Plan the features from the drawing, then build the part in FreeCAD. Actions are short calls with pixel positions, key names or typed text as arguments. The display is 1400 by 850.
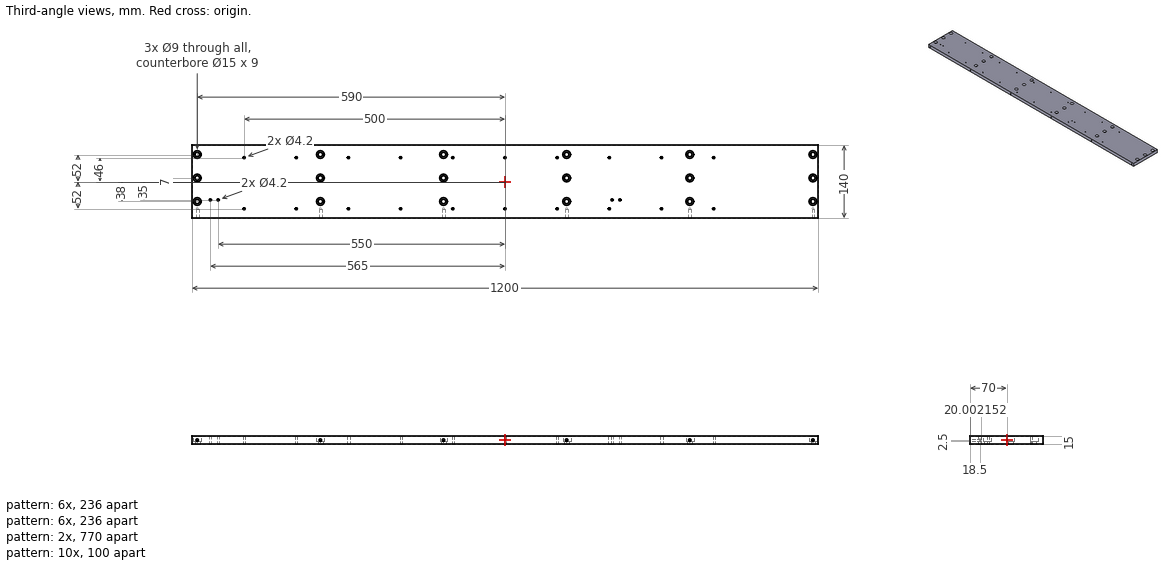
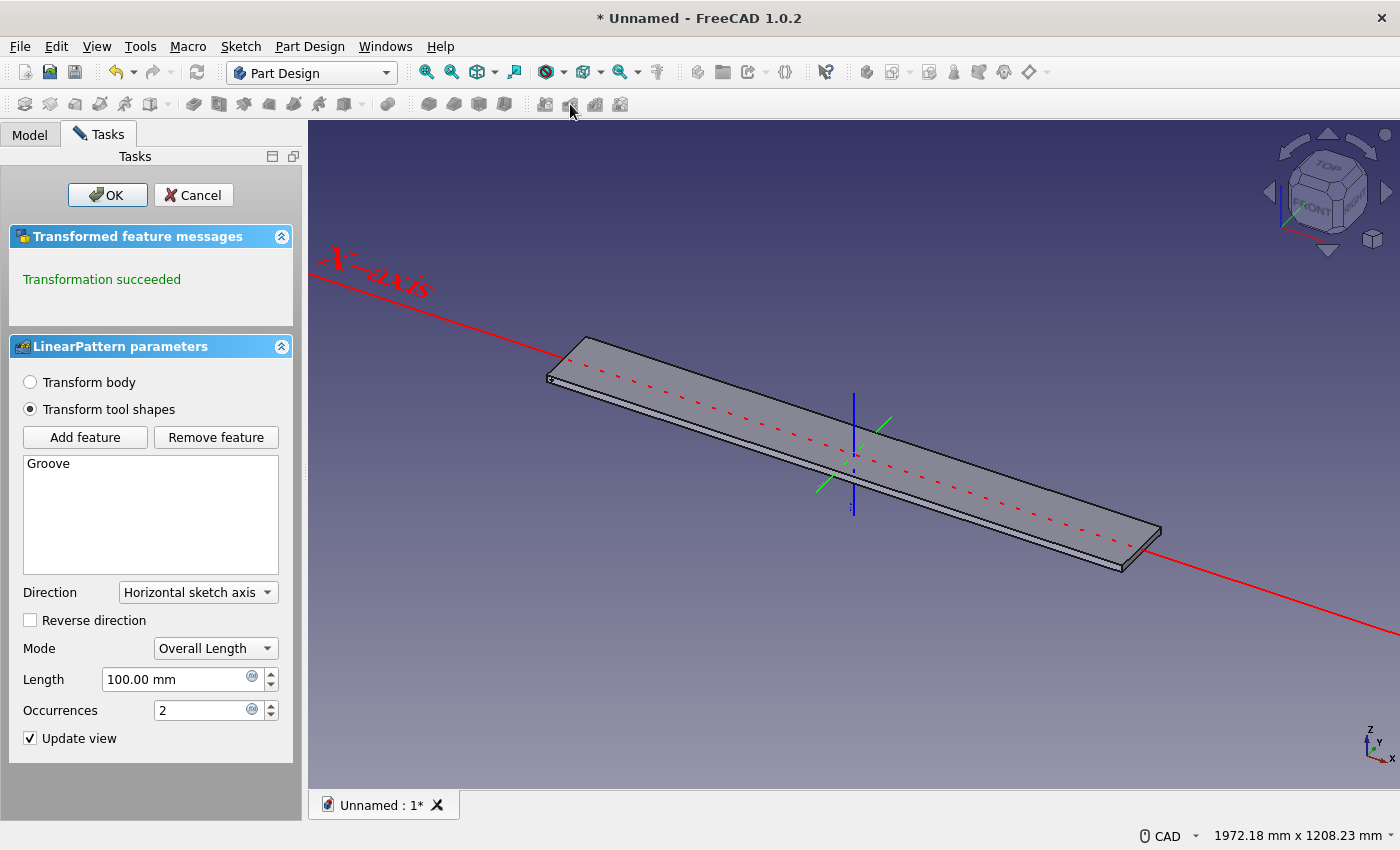
click(199, 592)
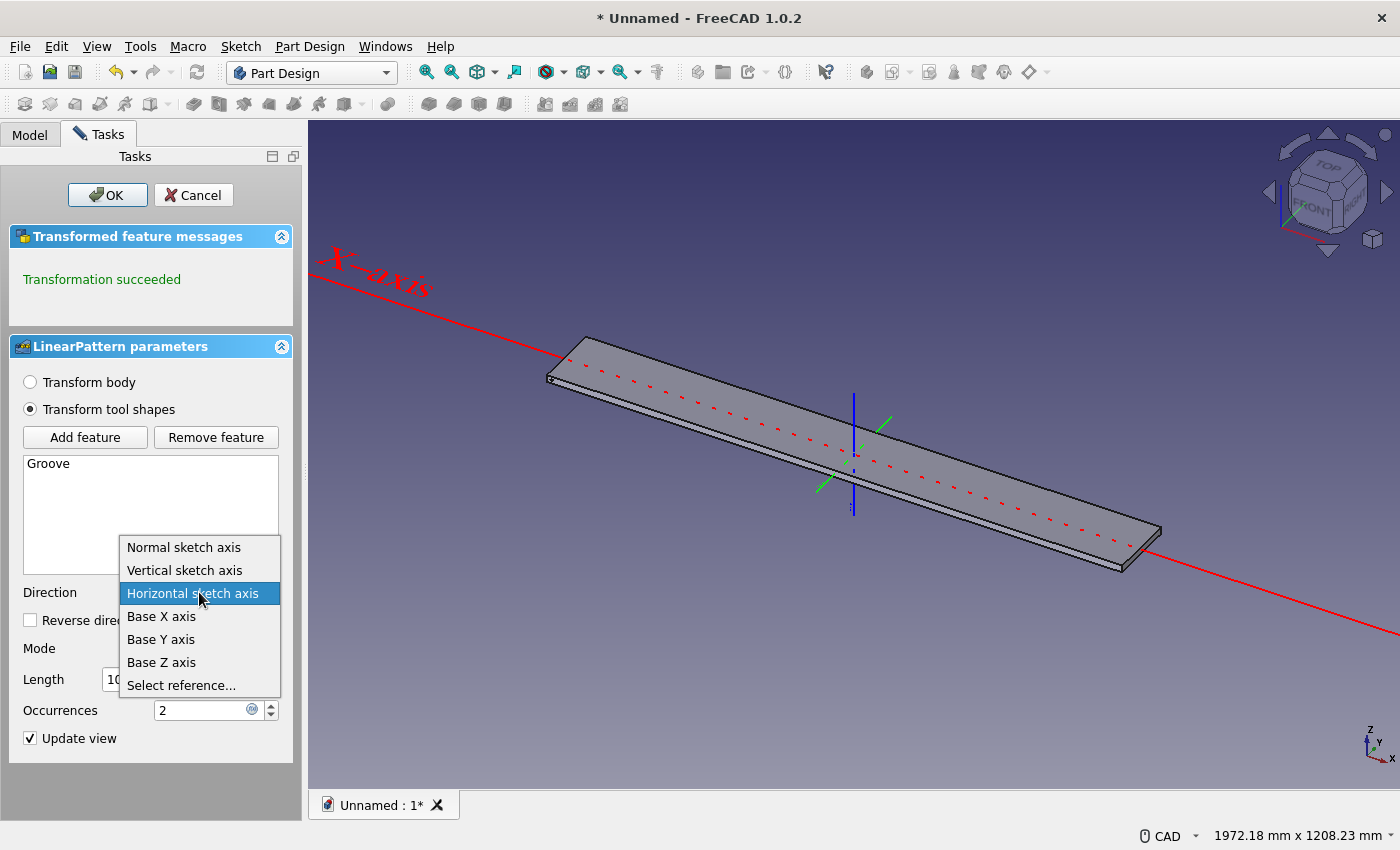
click(198, 616)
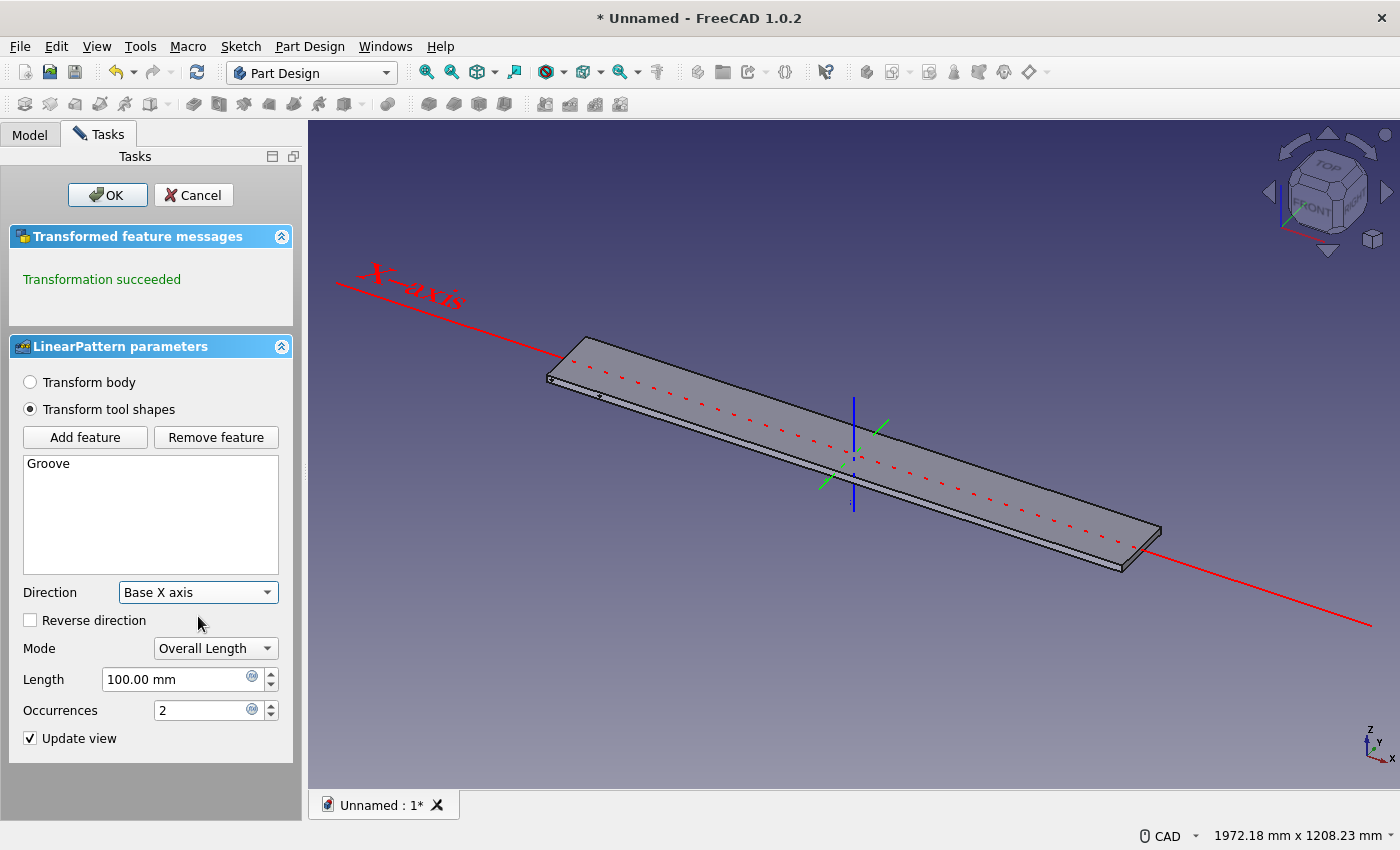
click(216, 648)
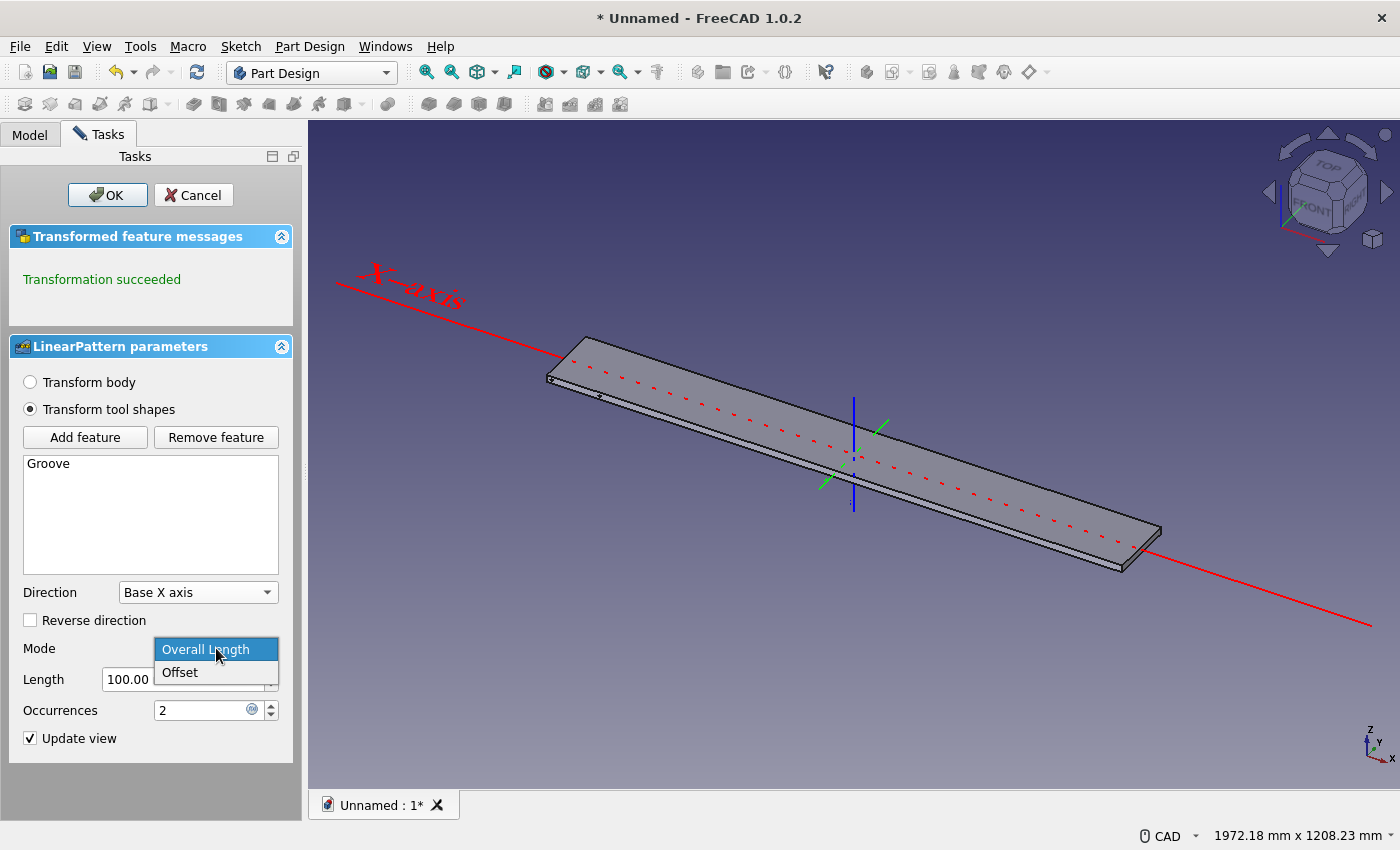
click(214, 672)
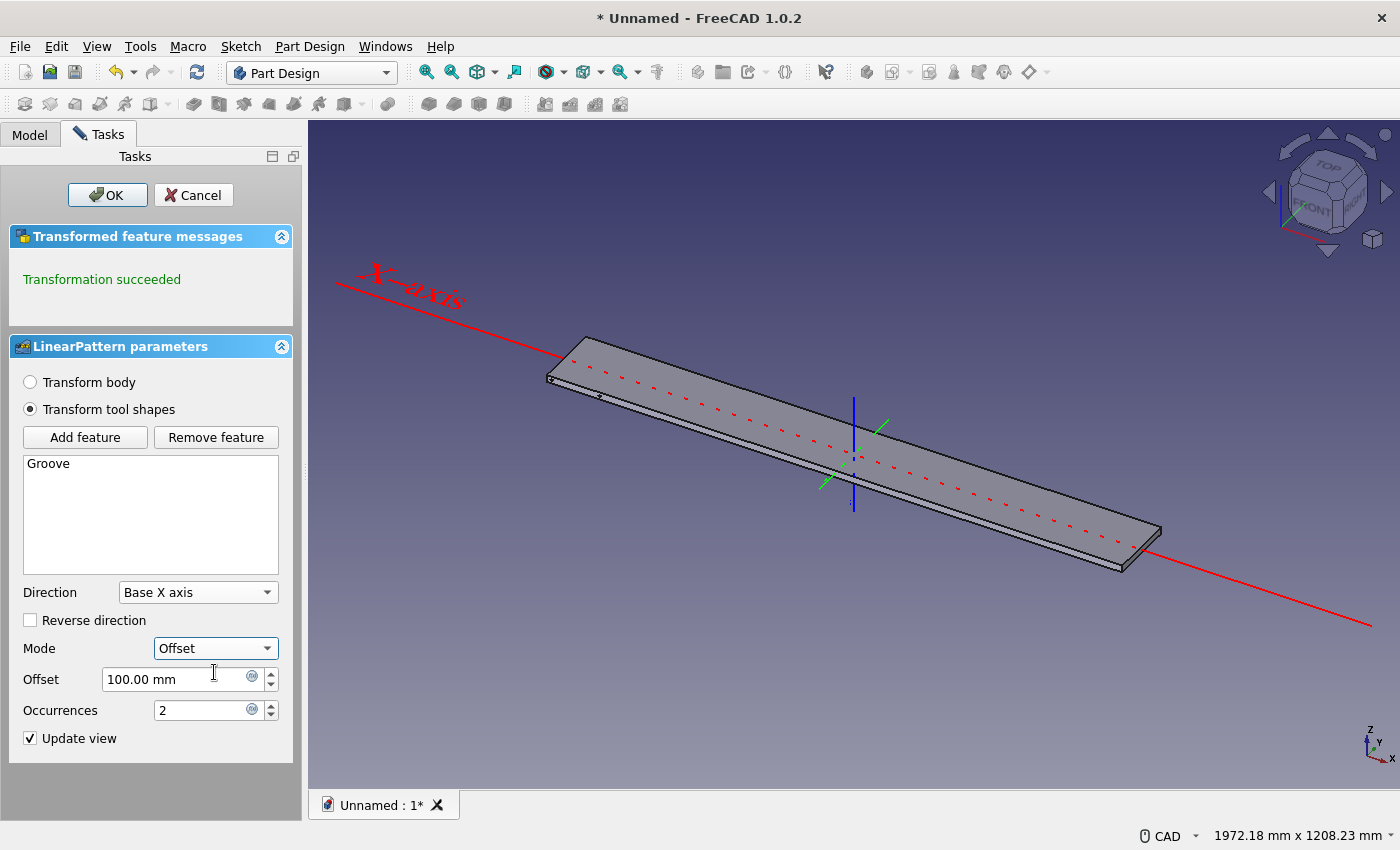
triple_click(184, 680)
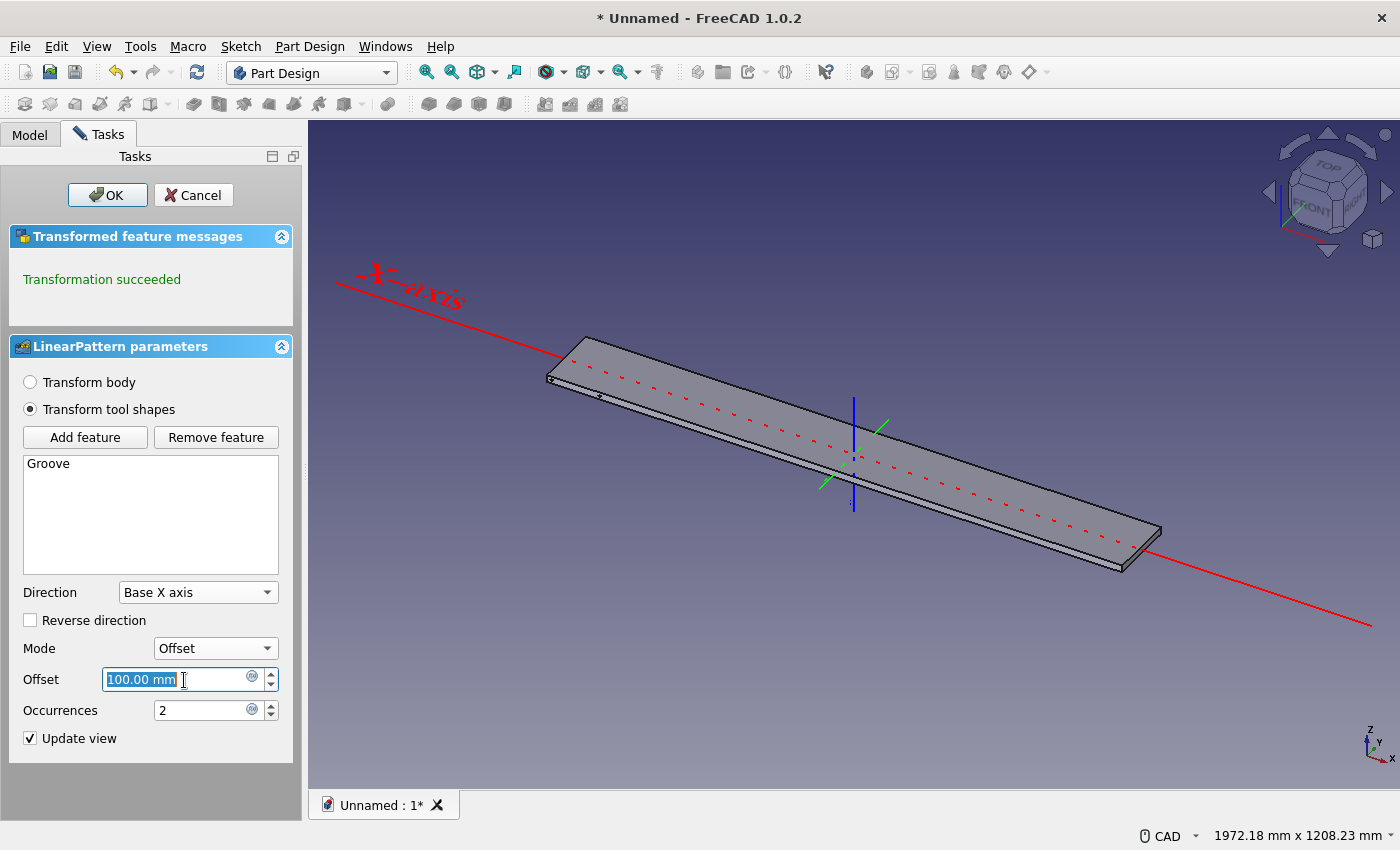
text(236)
key(Tab)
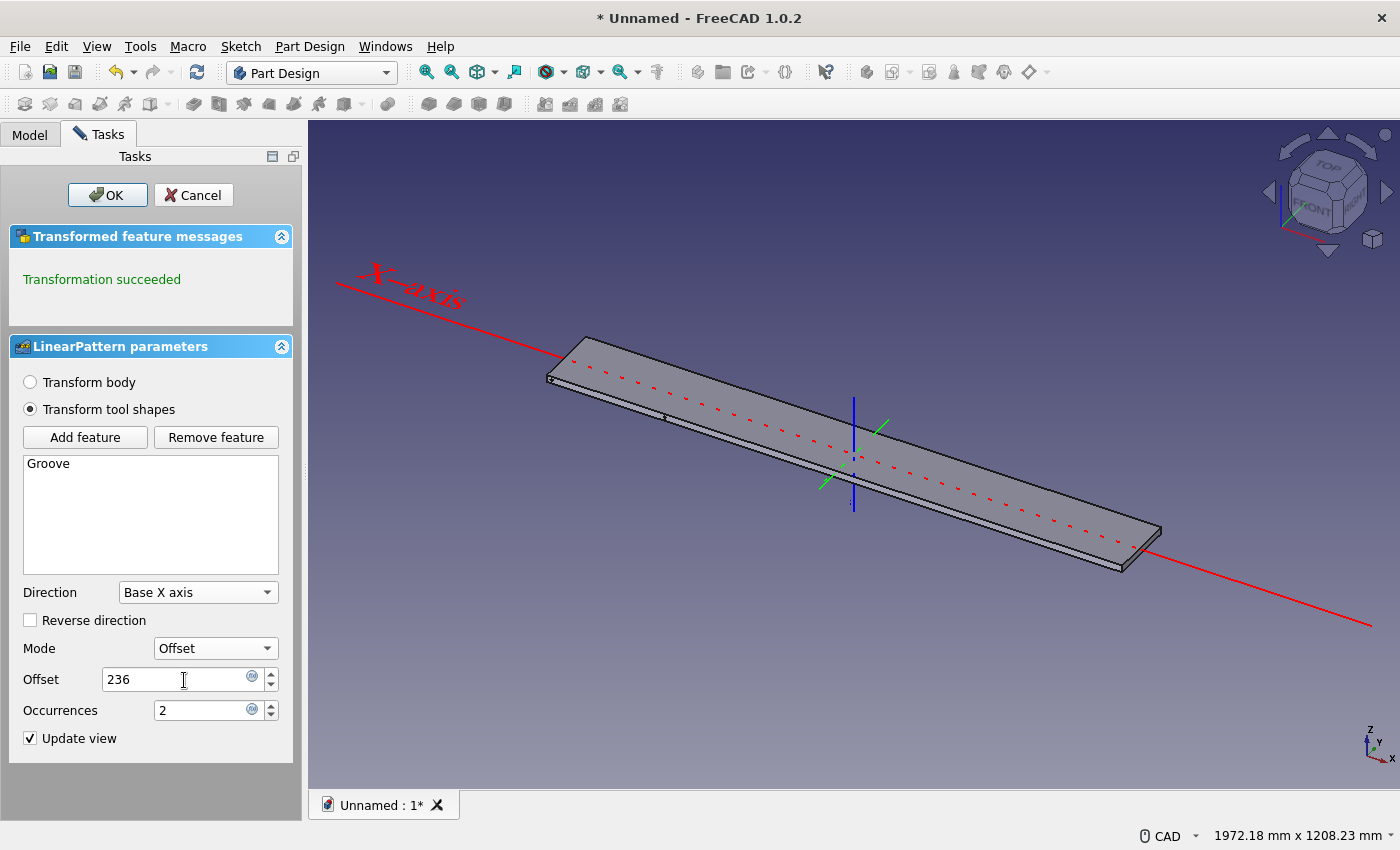
triple_click(210, 710)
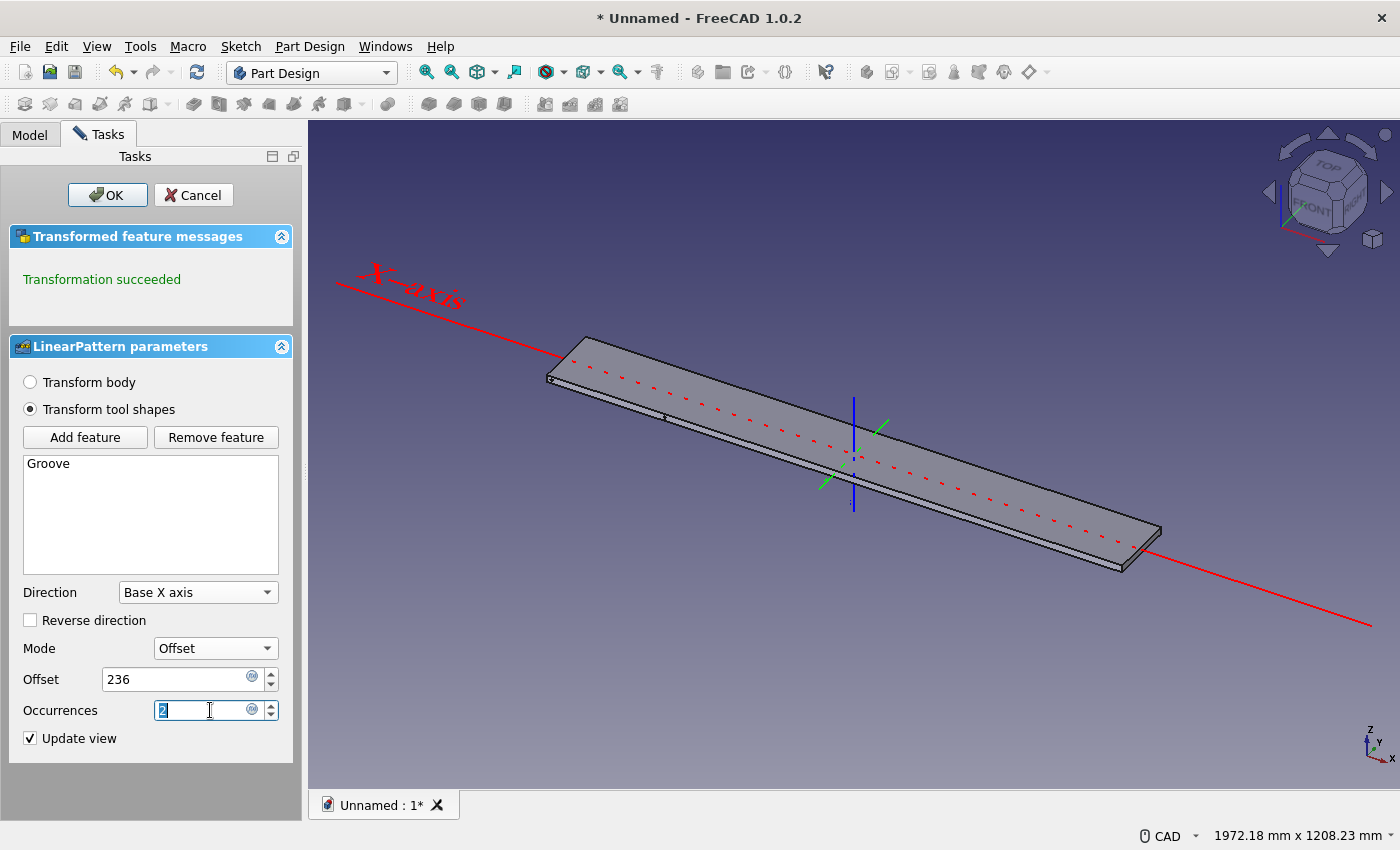
text(6)
key(Tab)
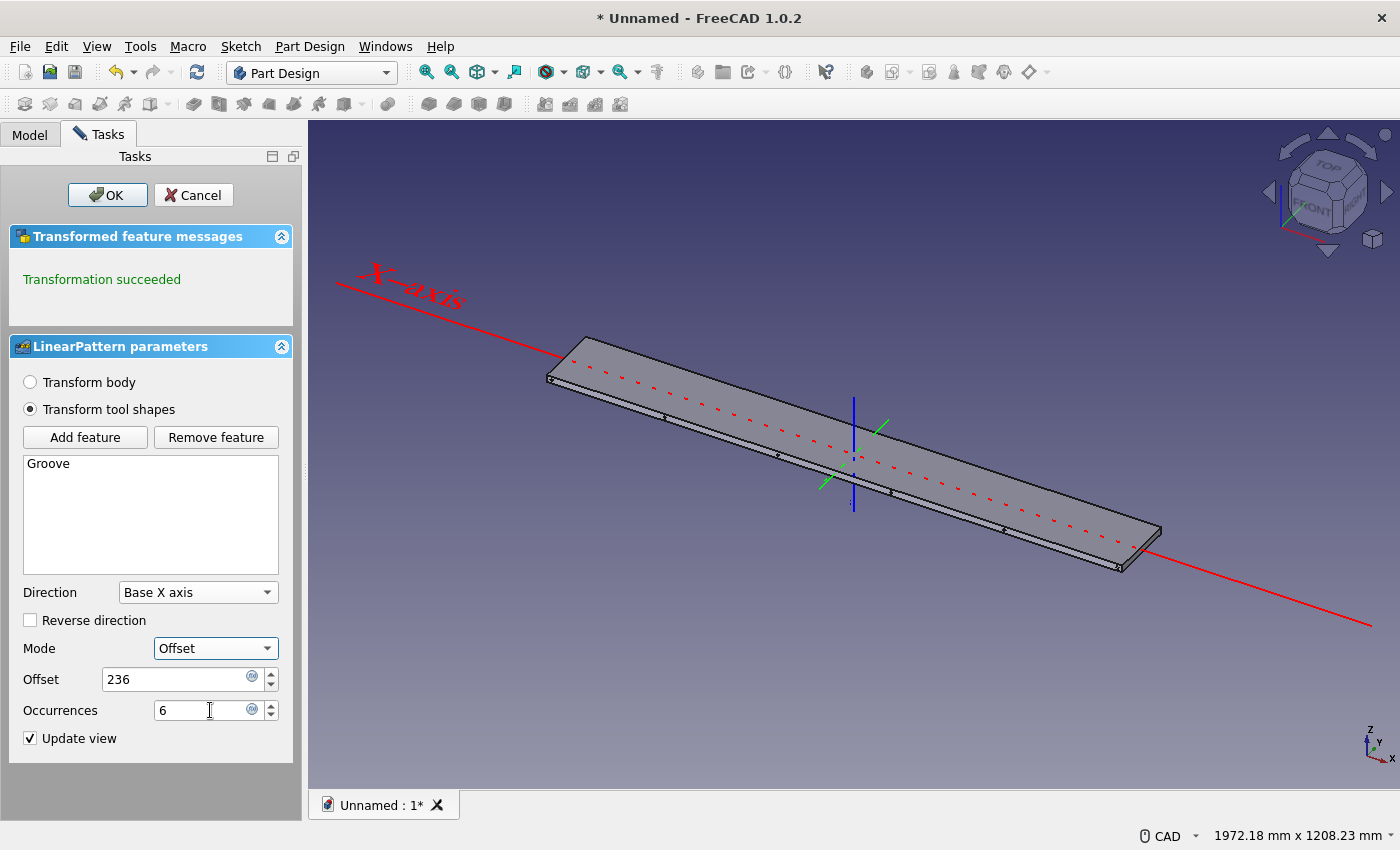
click(108, 195)